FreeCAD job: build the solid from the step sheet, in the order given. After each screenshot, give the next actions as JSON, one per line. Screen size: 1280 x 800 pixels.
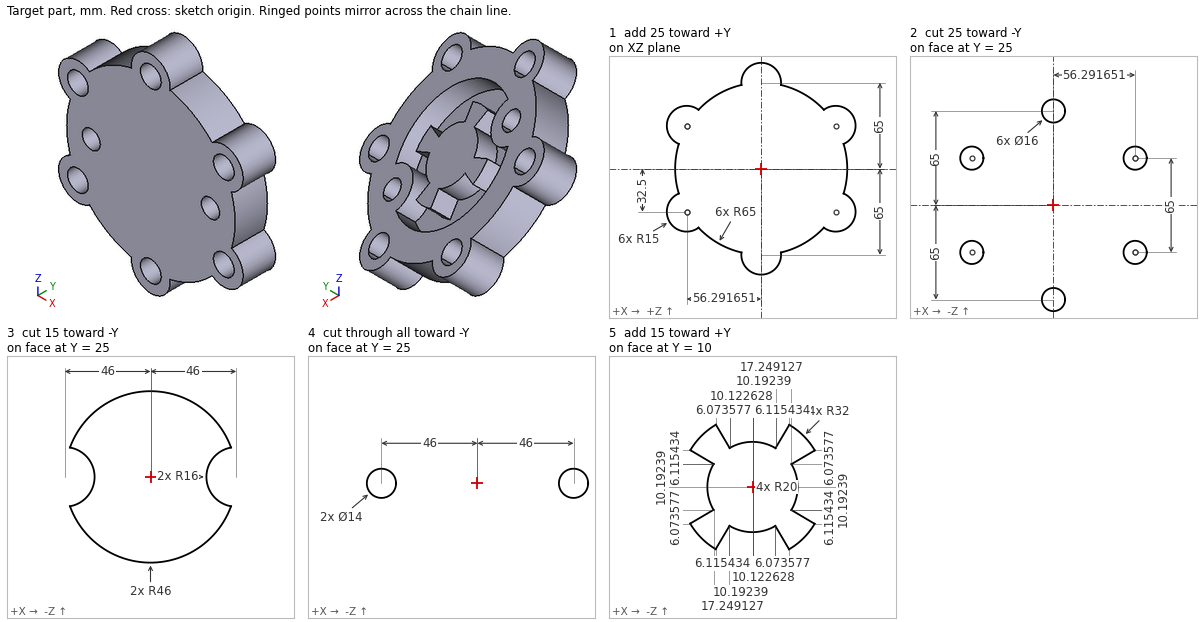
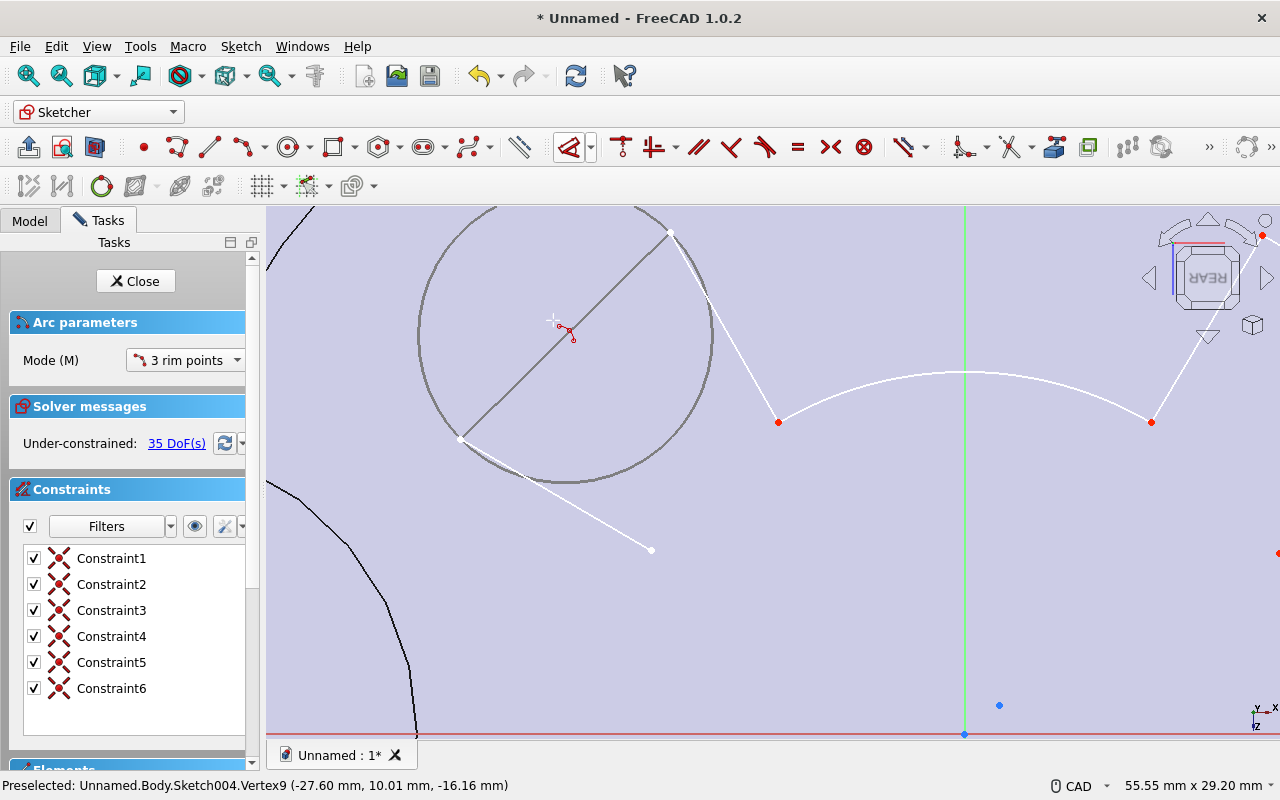
{"action": "left_click", "coordinate": [552, 320]}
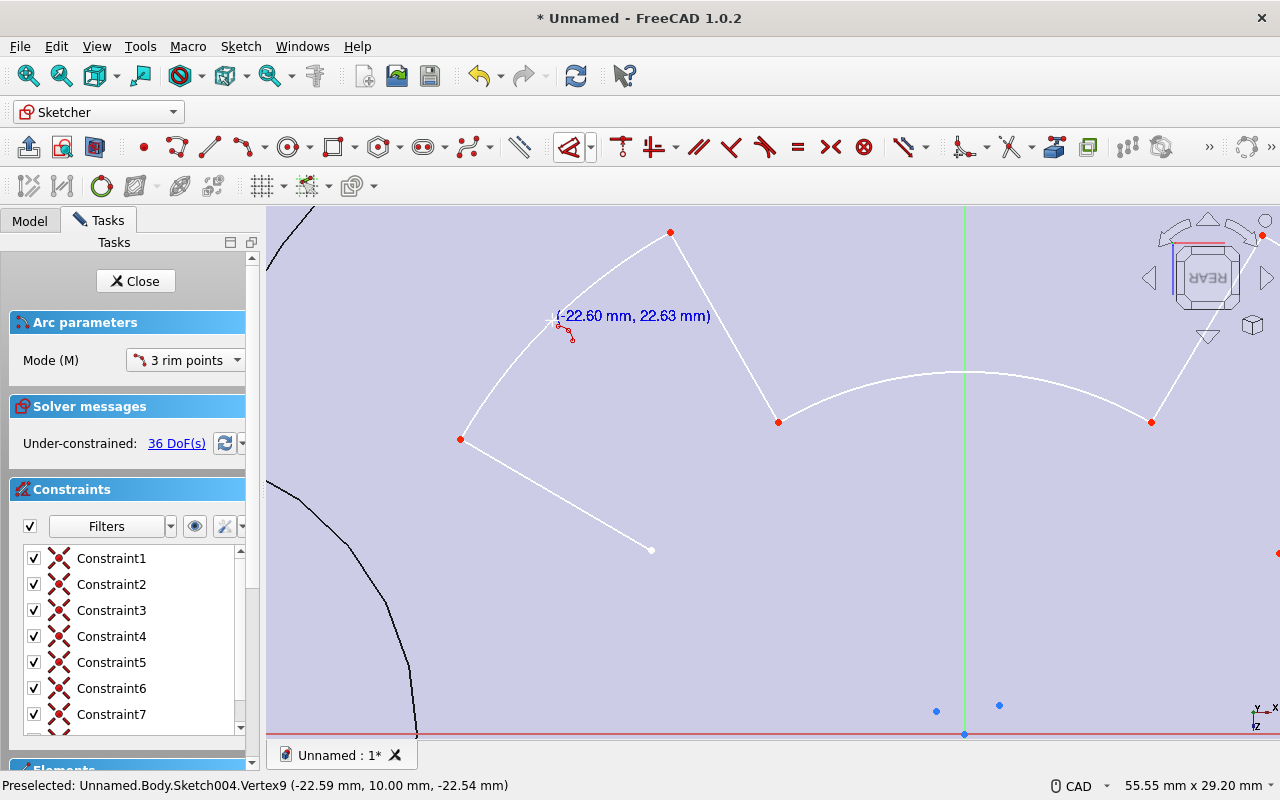
{"action": "left_click", "coordinate": [651, 551]}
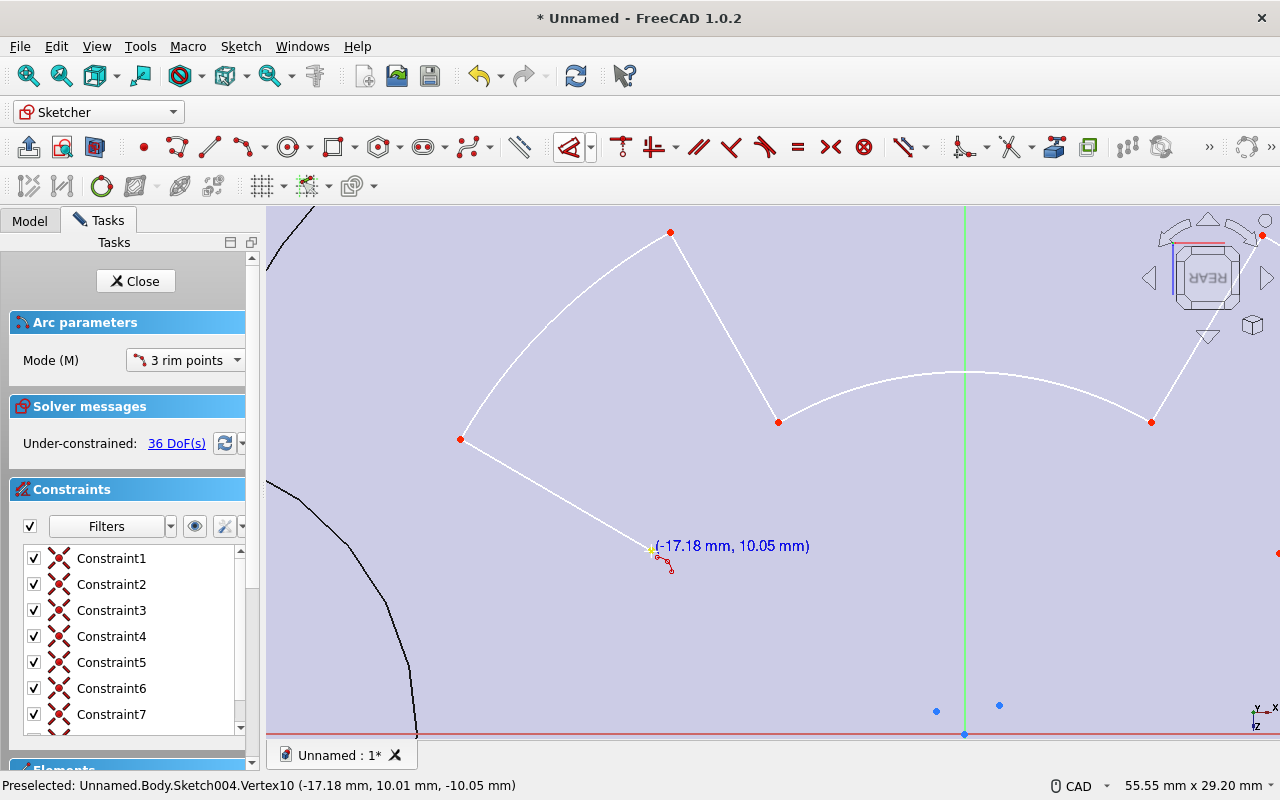
{"action": "scroll", "coordinate": [553, 320], "scroll_direction": "down", "scroll_amount": 5}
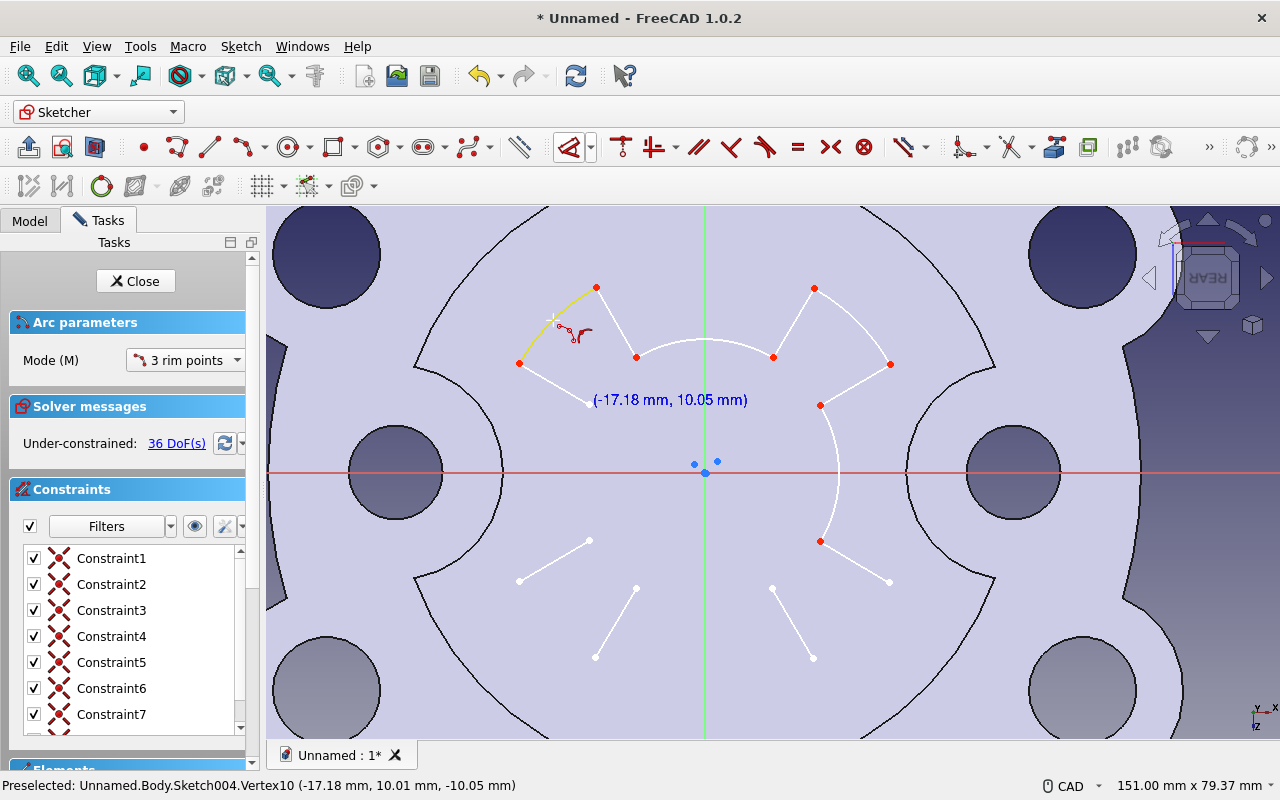
{"action": "left_click", "coordinate": [589, 541]}
{"action": "left_click", "coordinate": [571, 458]}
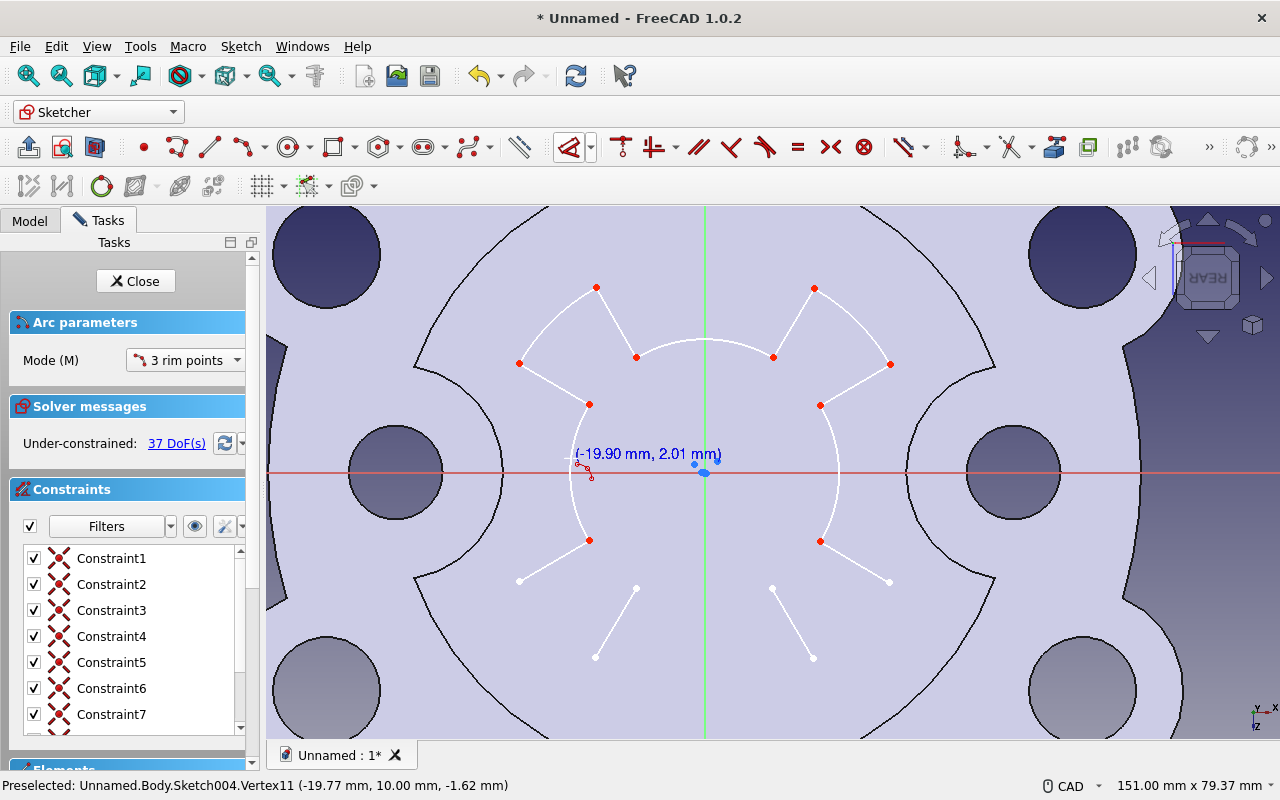
{"action": "left_click", "coordinate": [519, 582]}
{"action": "left_click", "coordinate": [595, 658]}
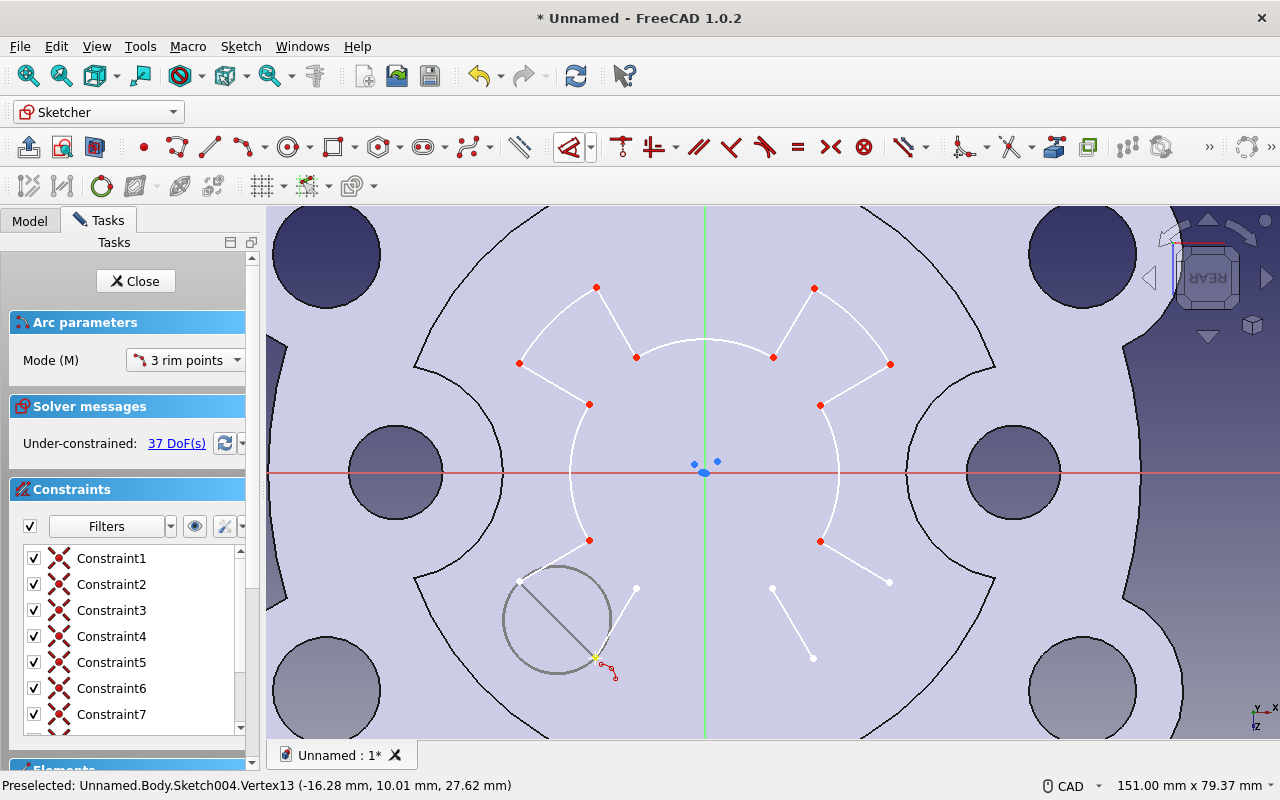
{"action": "scroll", "coordinate": [552, 624], "scroll_direction": "up", "scroll_amount": 5}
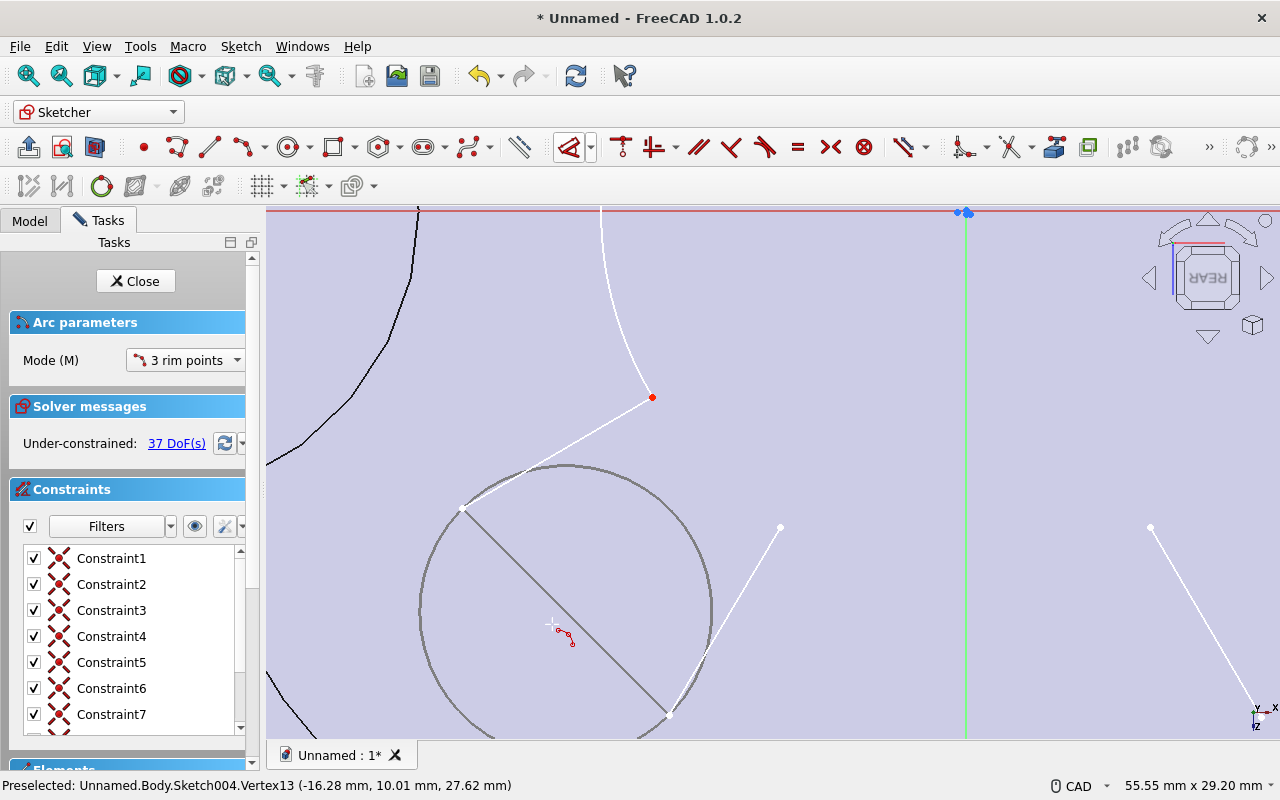
{"action": "left_click", "coordinate": [552, 623]}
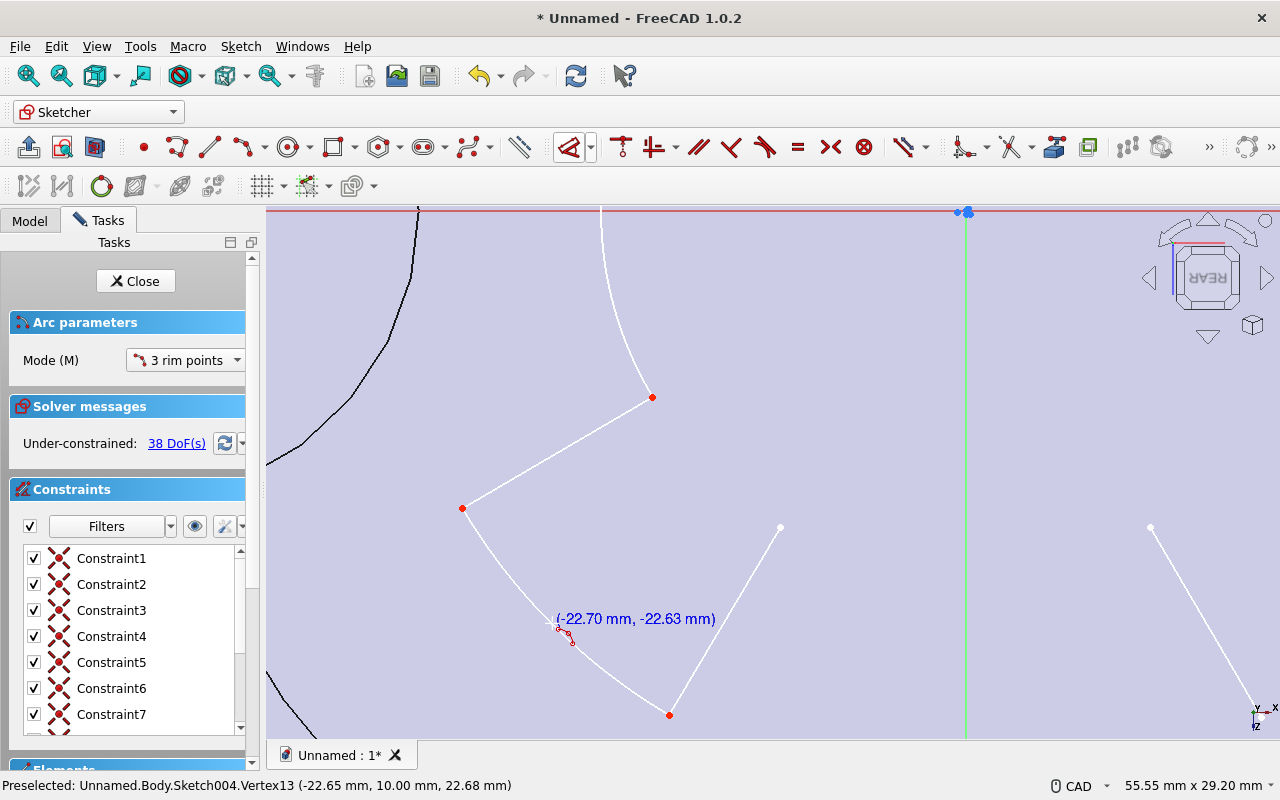
{"action": "left_click", "coordinate": [781, 528]}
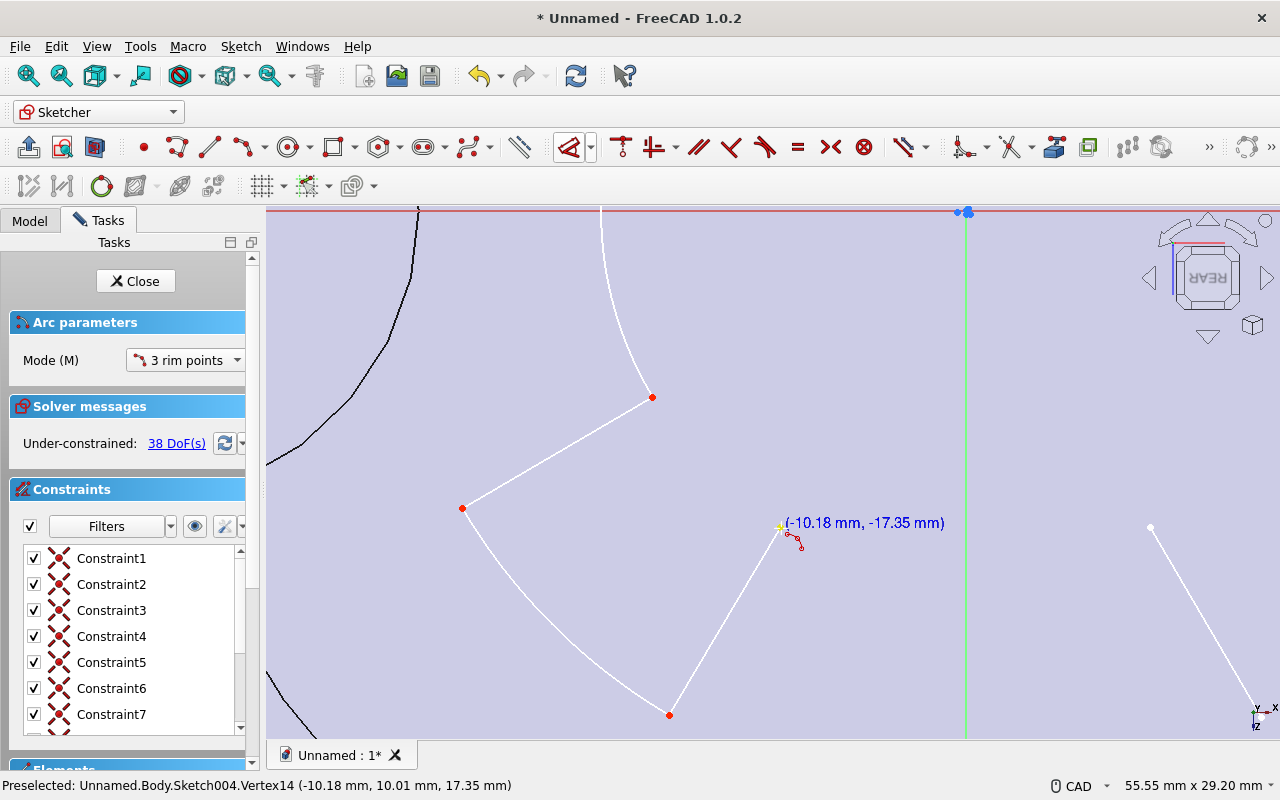
{"action": "scroll", "coordinate": [552, 625], "scroll_direction": "down", "scroll_amount": 5}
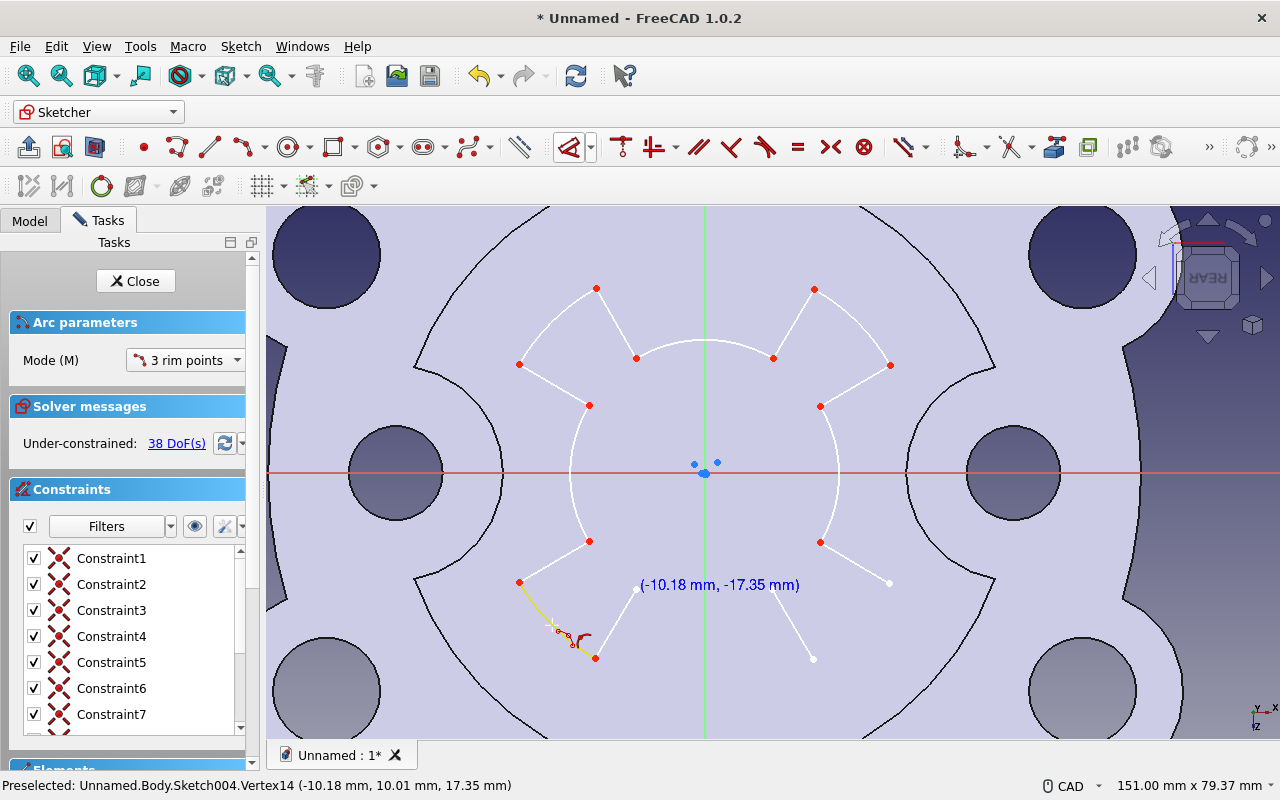
{"action": "left_click", "coordinate": [772, 590]}
{"action": "left_click", "coordinate": [690, 607]}